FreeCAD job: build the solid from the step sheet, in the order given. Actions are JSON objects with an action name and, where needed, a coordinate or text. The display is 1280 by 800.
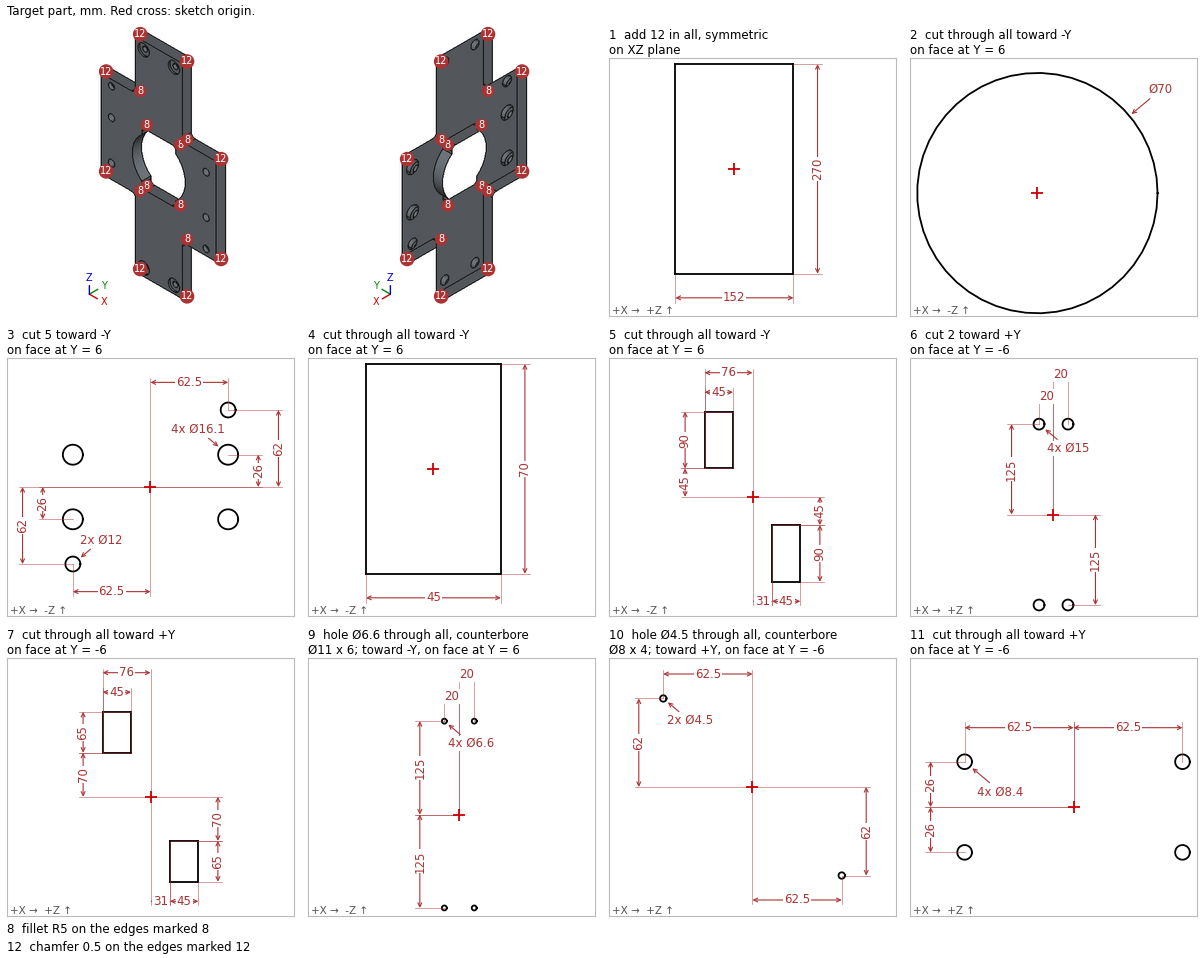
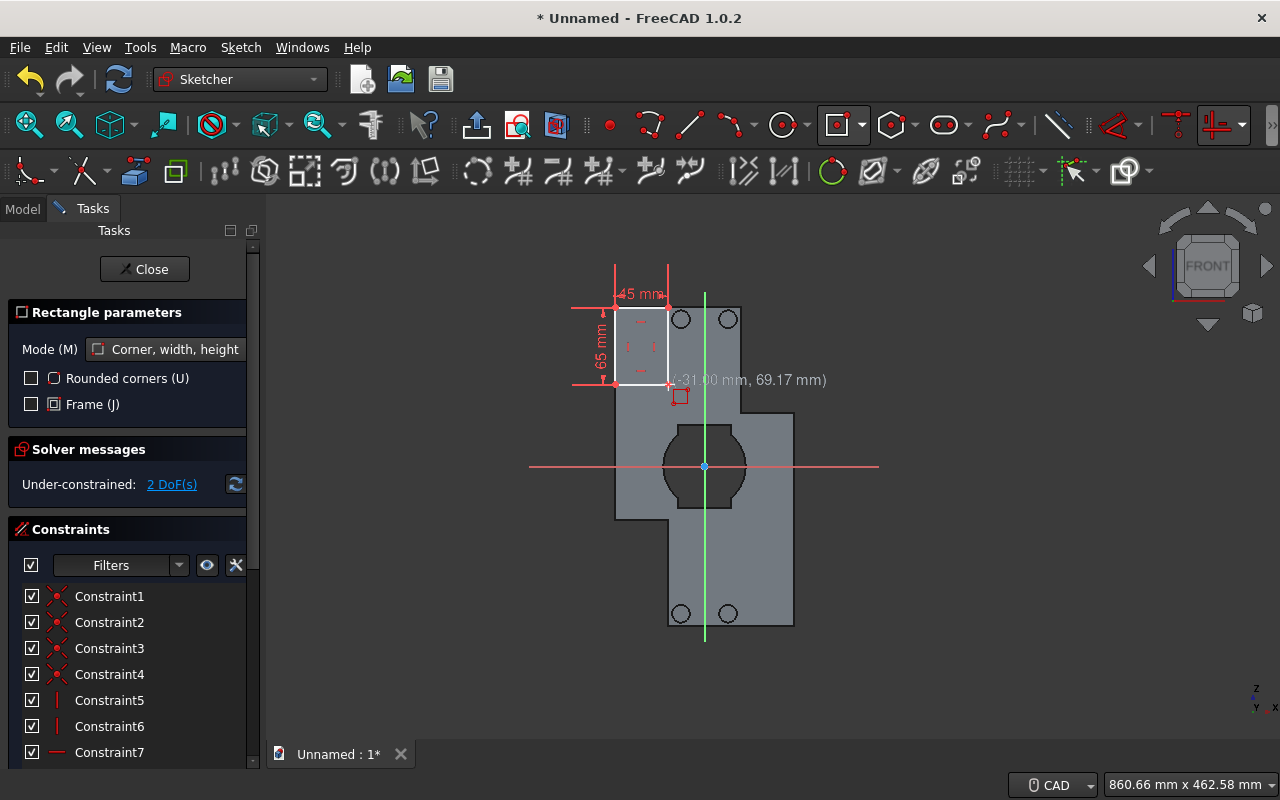
{"action": "left_click", "coordinate": [741, 549]}
{"action": "mouse_move", "coordinate": [794, 626]}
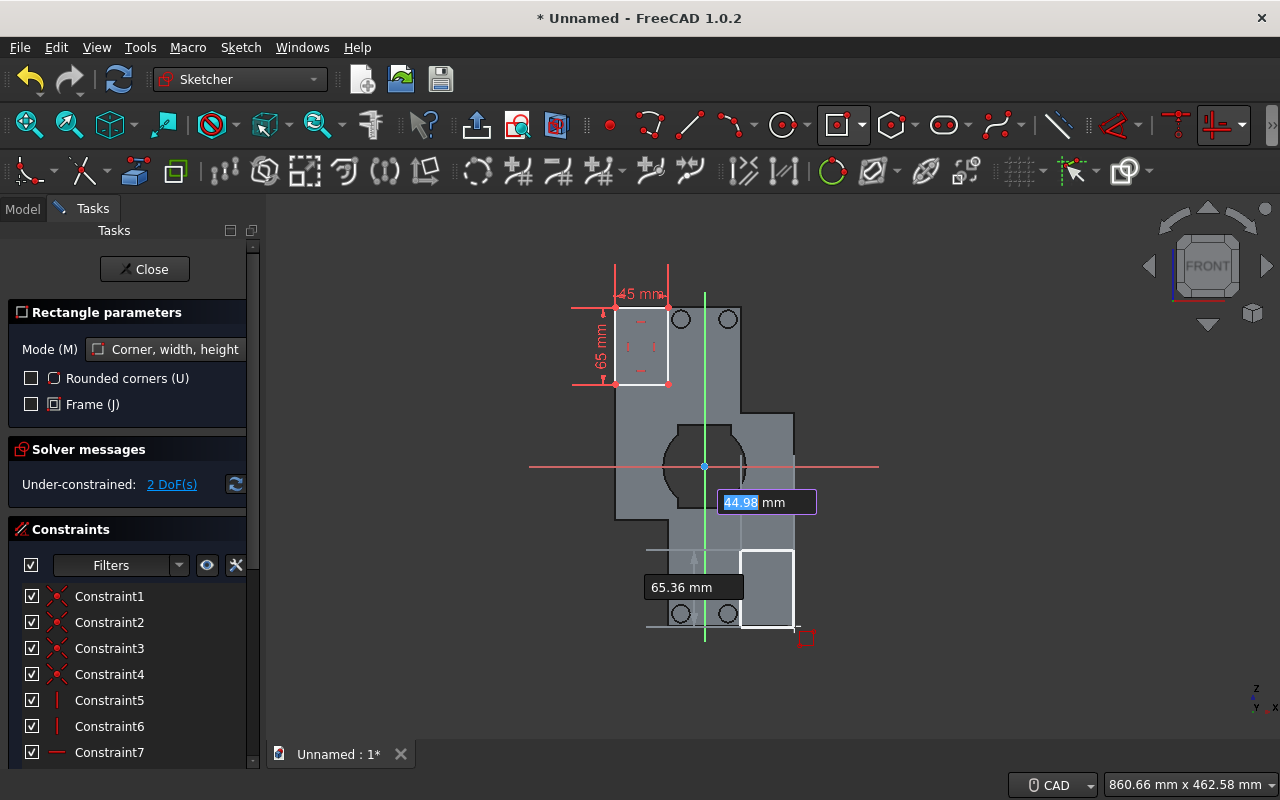
{"action": "type", "text": "45"}
{"action": "key", "text": "Tab"}
{"action": "type", "text": "65"}
{"action": "key", "text": "Return"}
{"action": "key", "text": "Escape"}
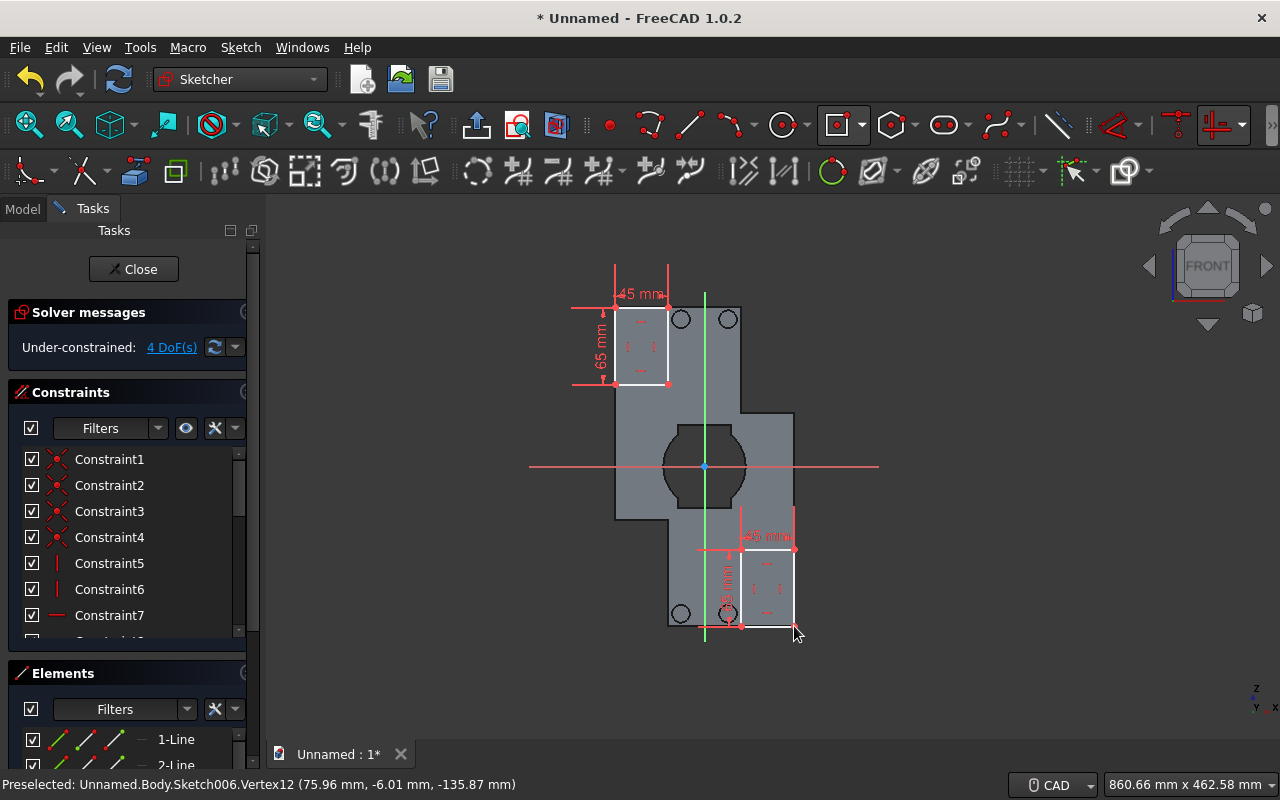
{"action": "key", "text": "d"}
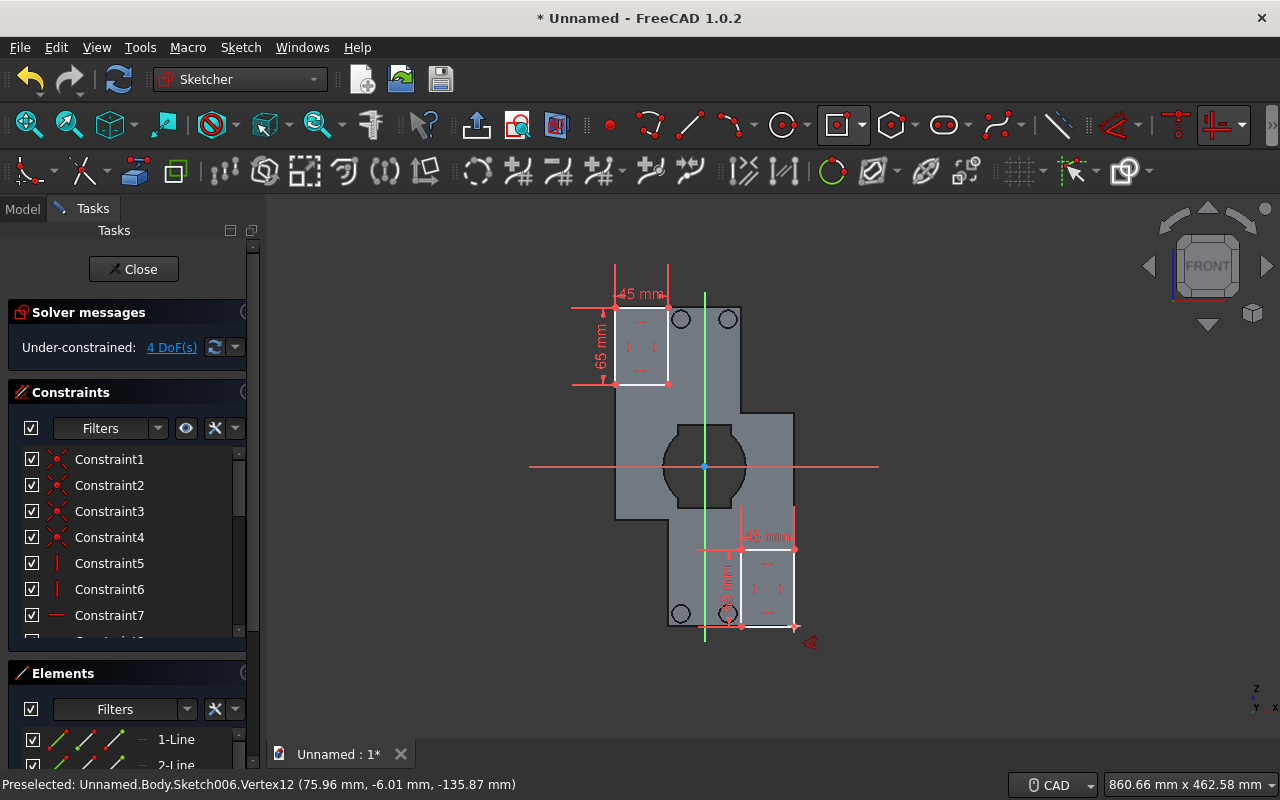
{"action": "left_click", "coordinate": [615, 308]}
{"action": "left_click", "coordinate": [660, 274]}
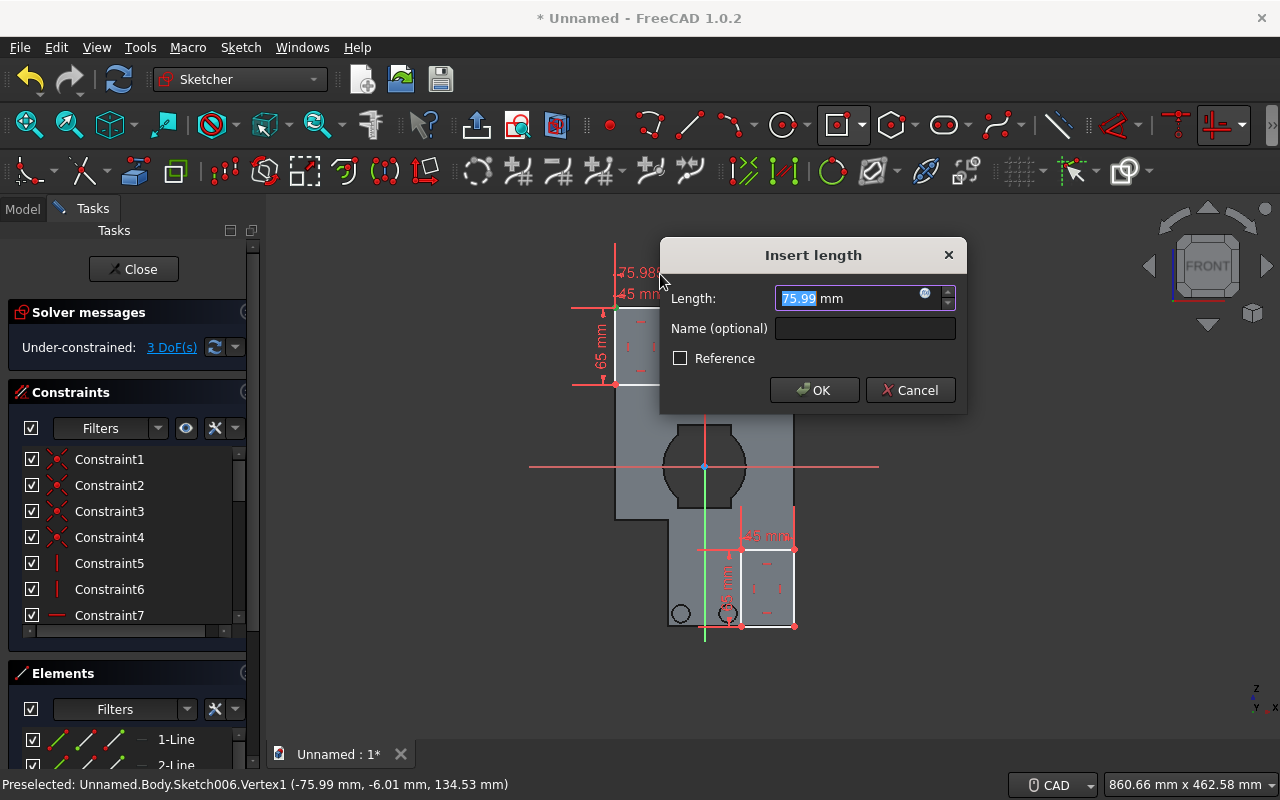
{"action": "type", "text": "76"}
{"action": "key", "text": "Return"}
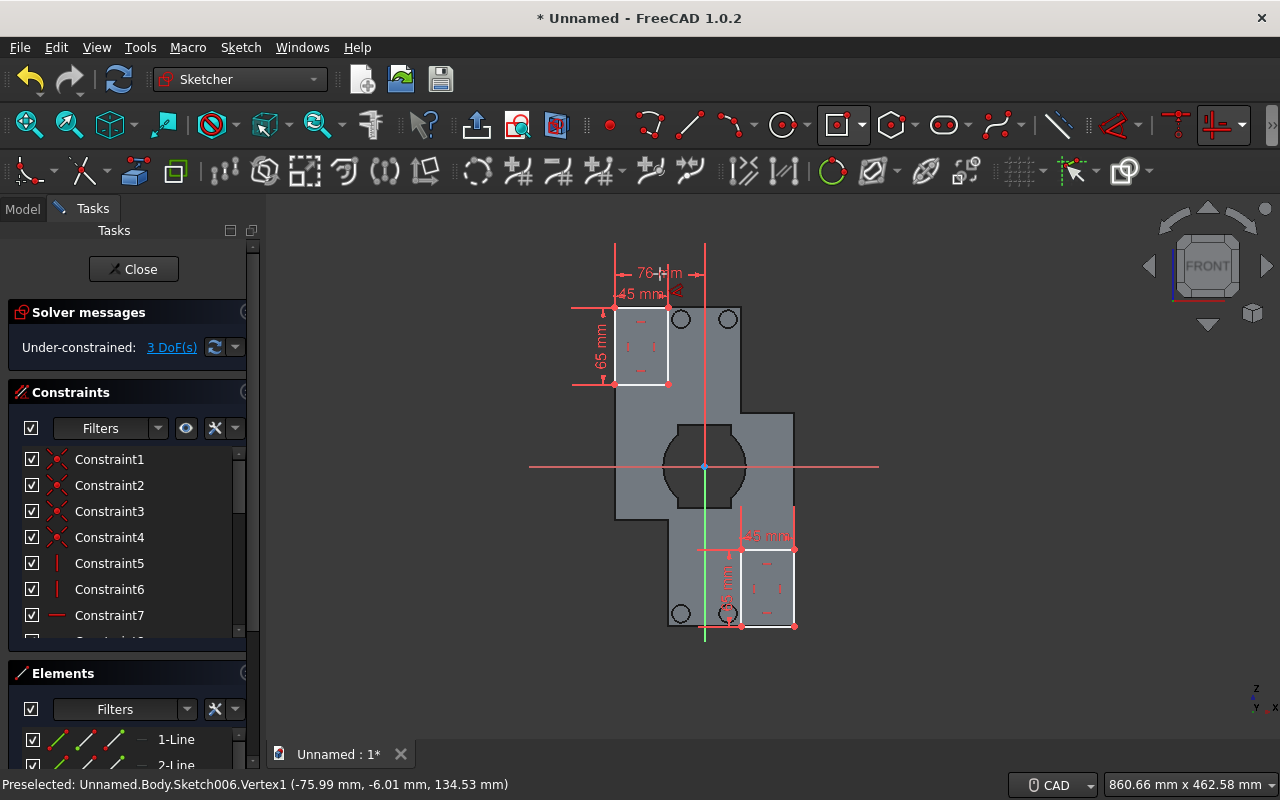
{"action": "left_click", "coordinate": [615, 385]}
{"action": "left_click", "coordinate": [581, 426]}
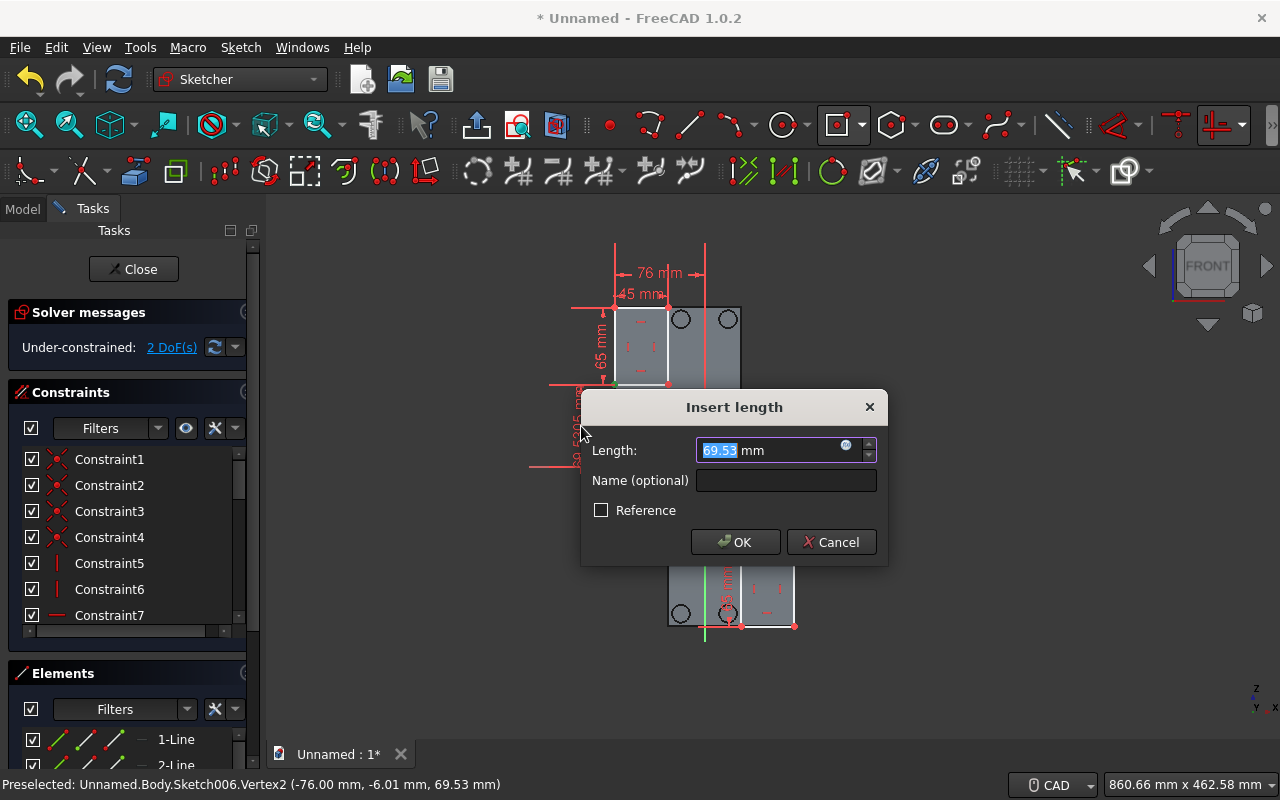
{"action": "type", "text": "70"}
{"action": "key", "text": "Return"}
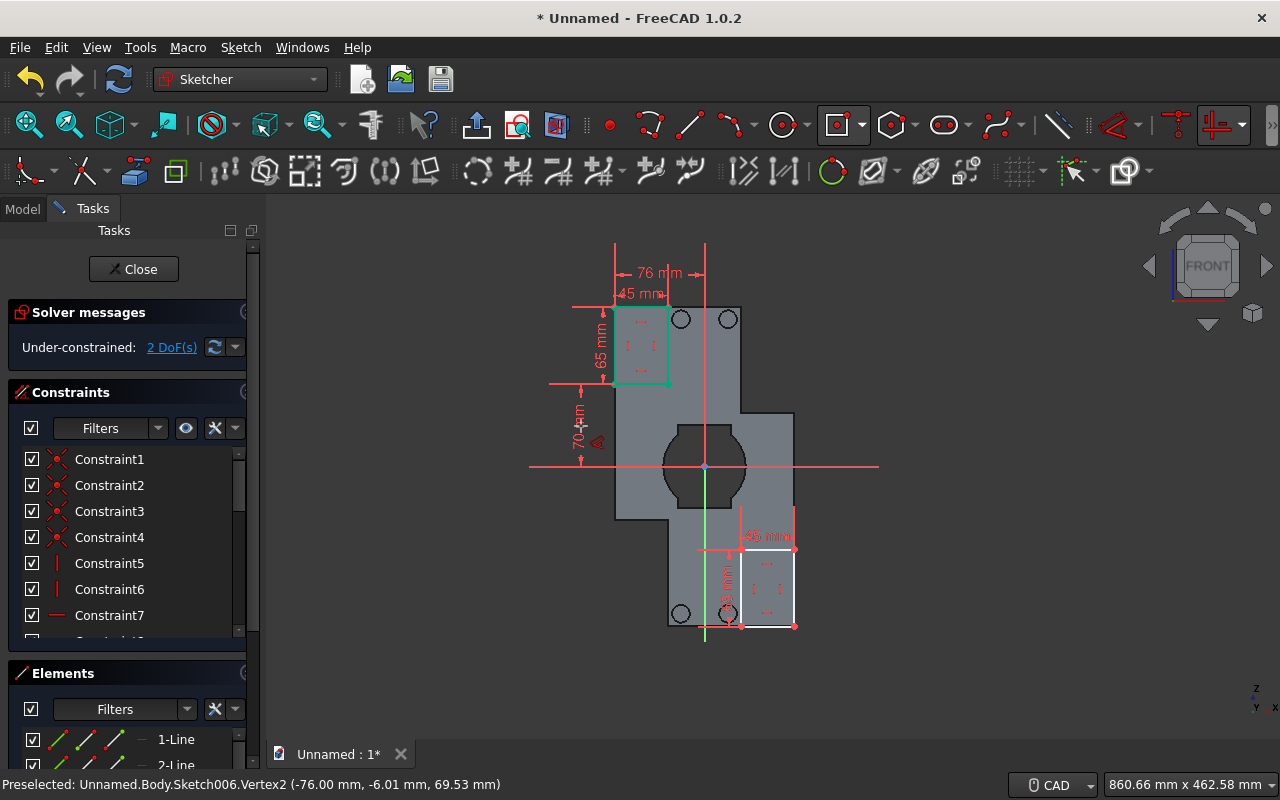
{"action": "left_click", "coordinate": [741, 550]}
{"action": "left_click", "coordinate": [723, 584]}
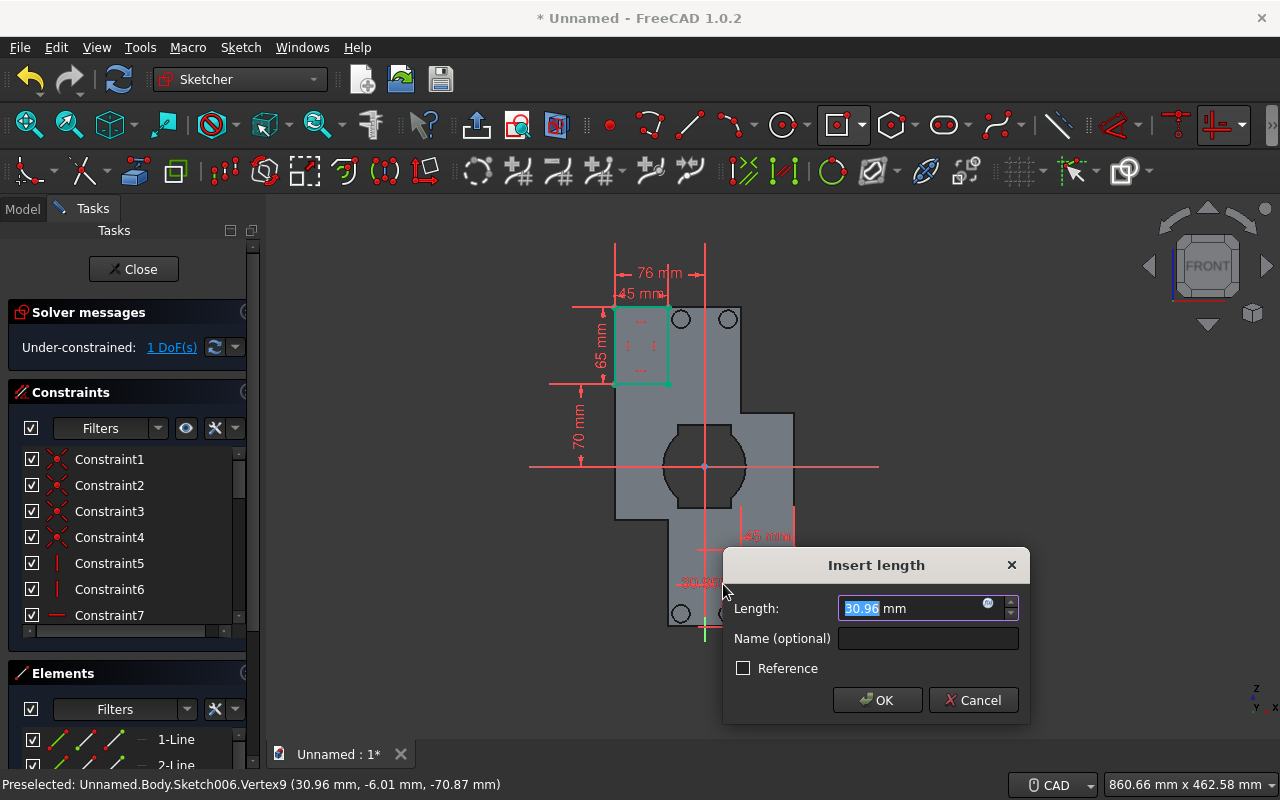
{"action": "type", "text": "31"}
{"action": "key", "text": "Return"}